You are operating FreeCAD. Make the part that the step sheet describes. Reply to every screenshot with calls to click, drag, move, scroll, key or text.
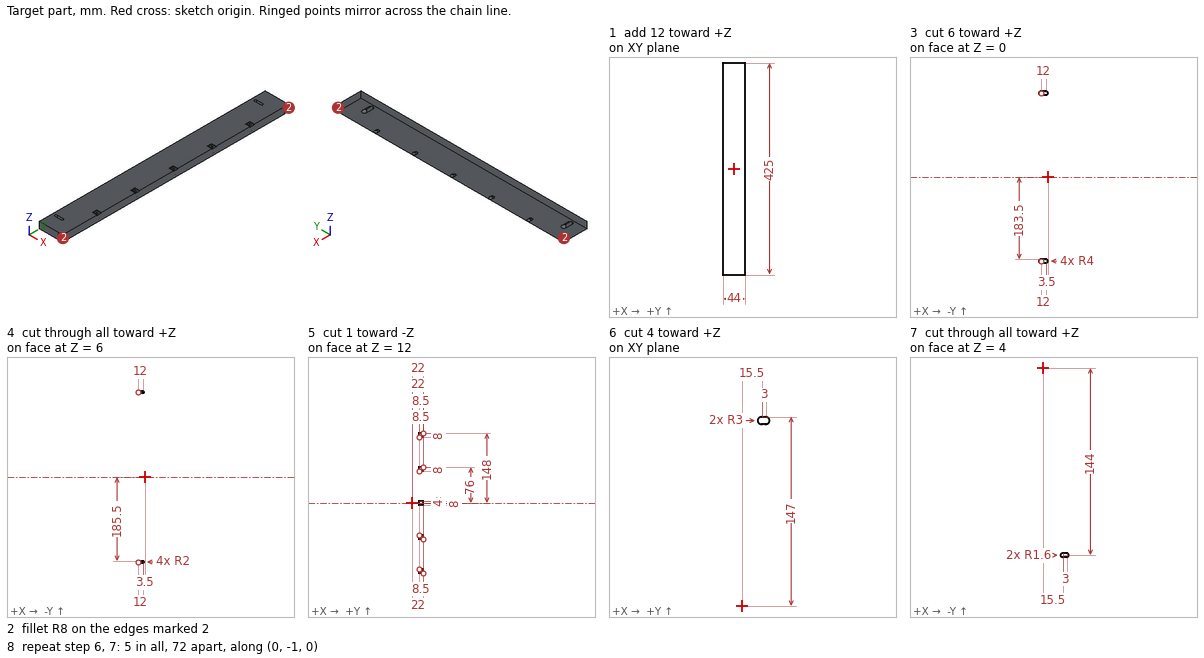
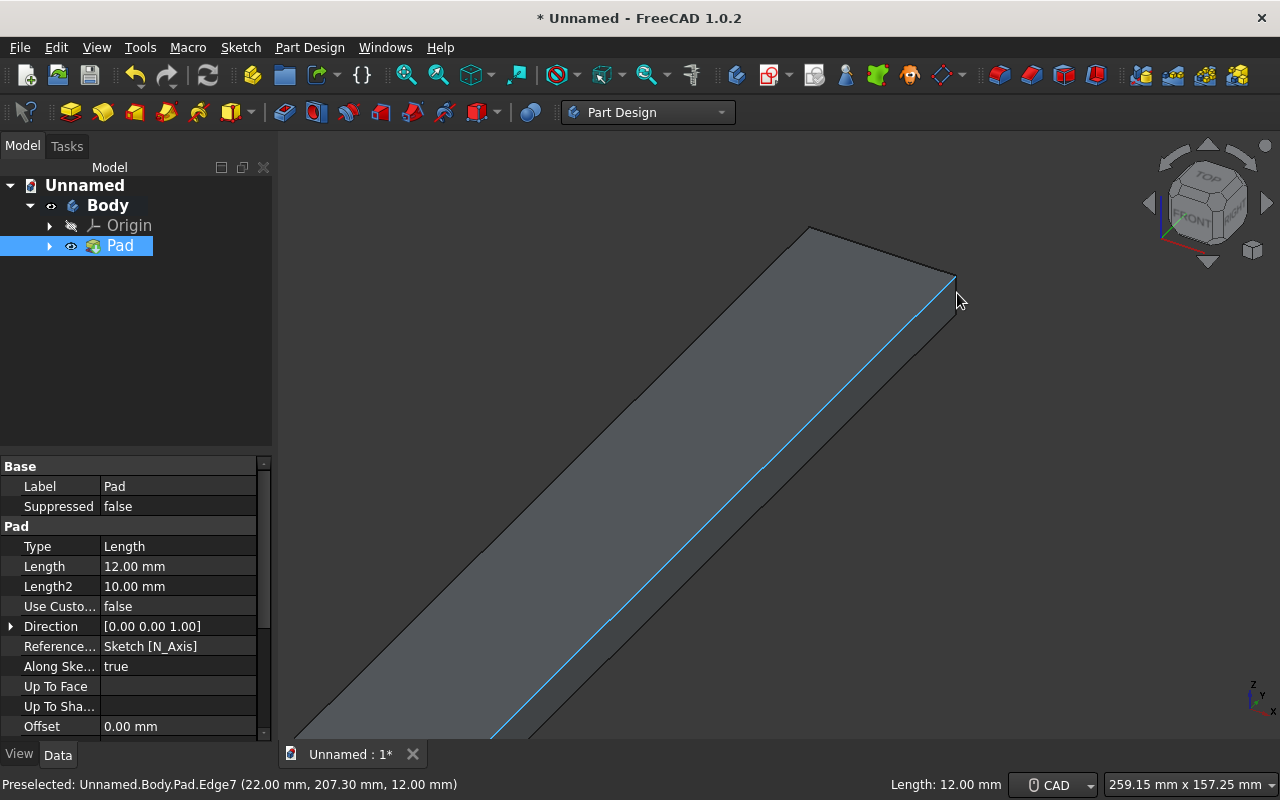
click(408, 76)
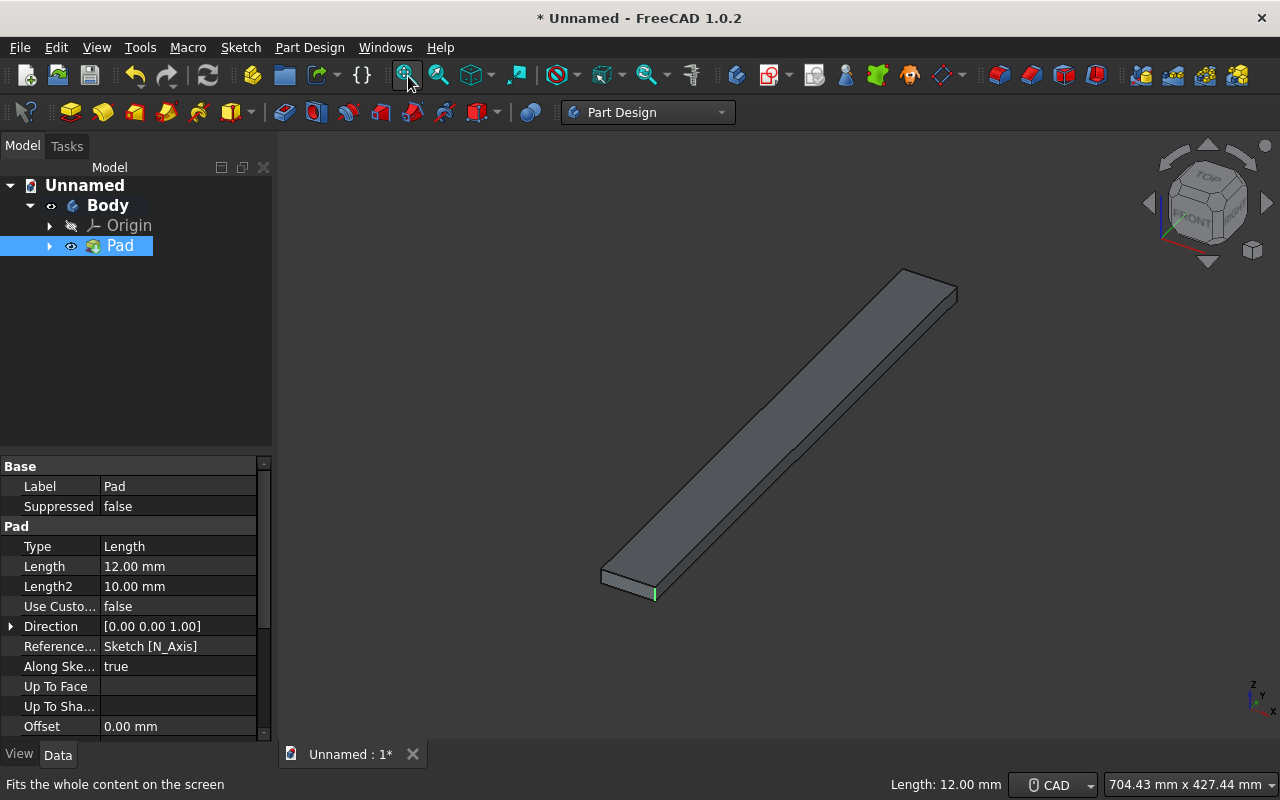
key(0)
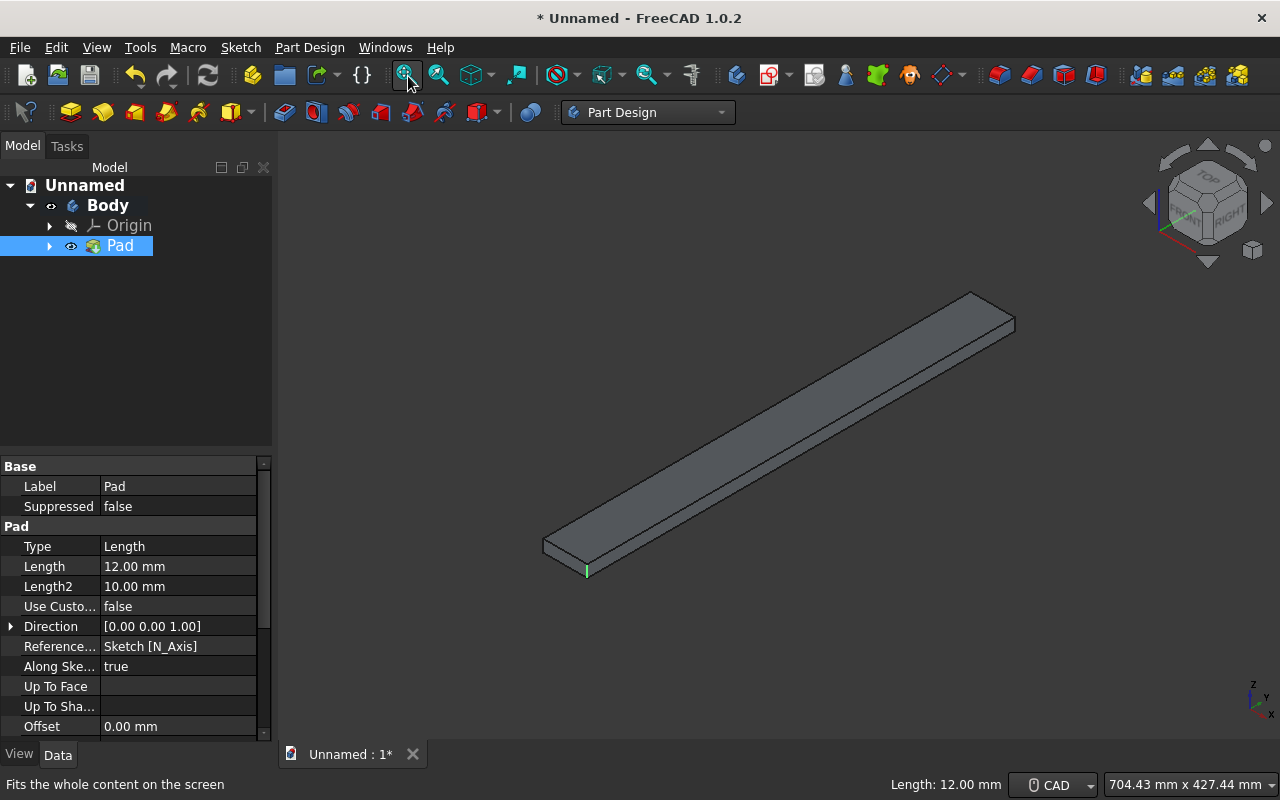
scroll(1015, 323, up, 5)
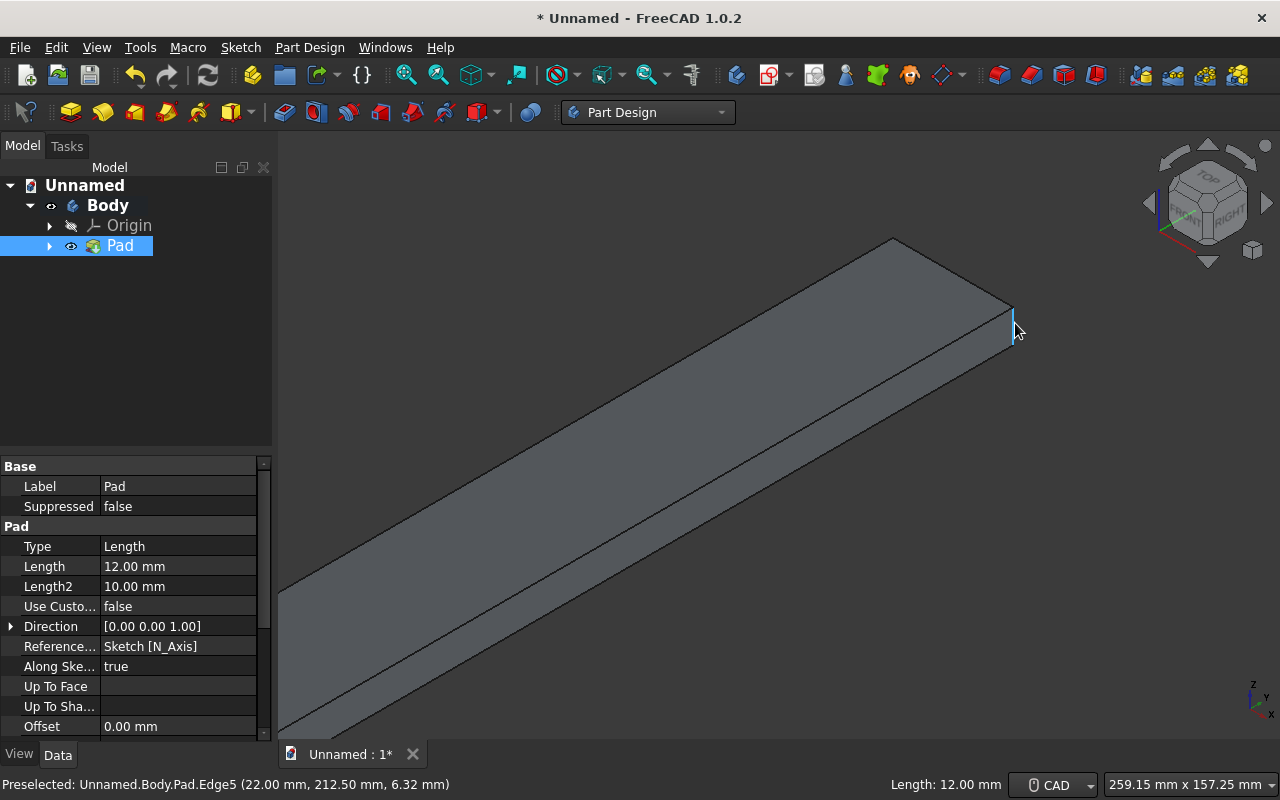
key(v)
key(f)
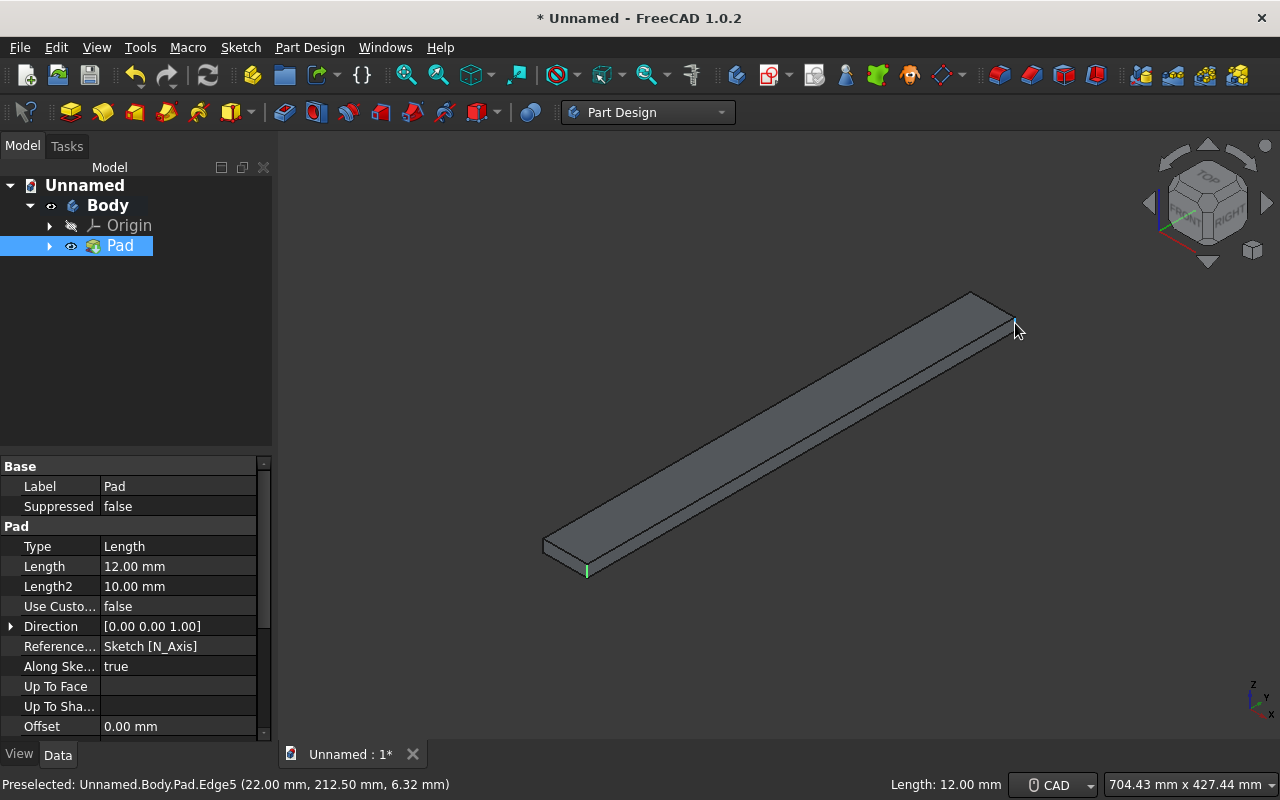
key(2)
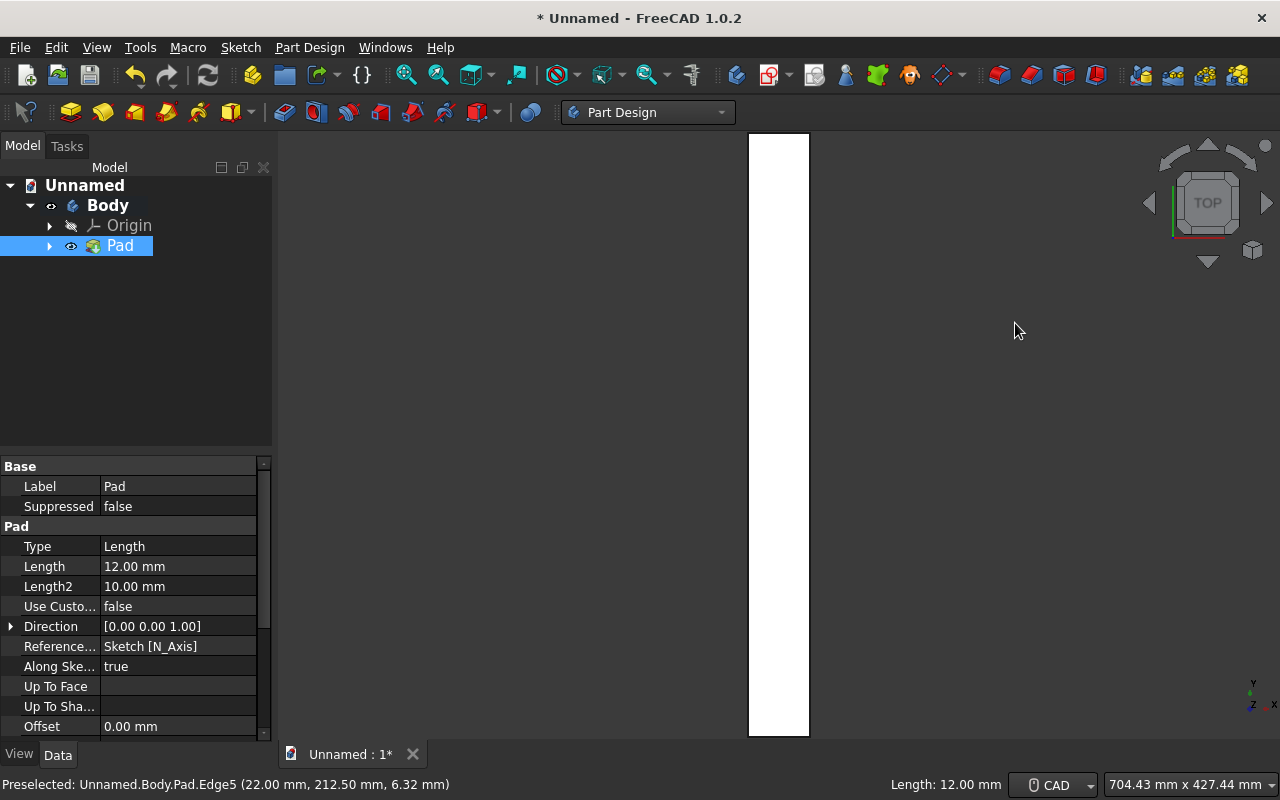
key(1)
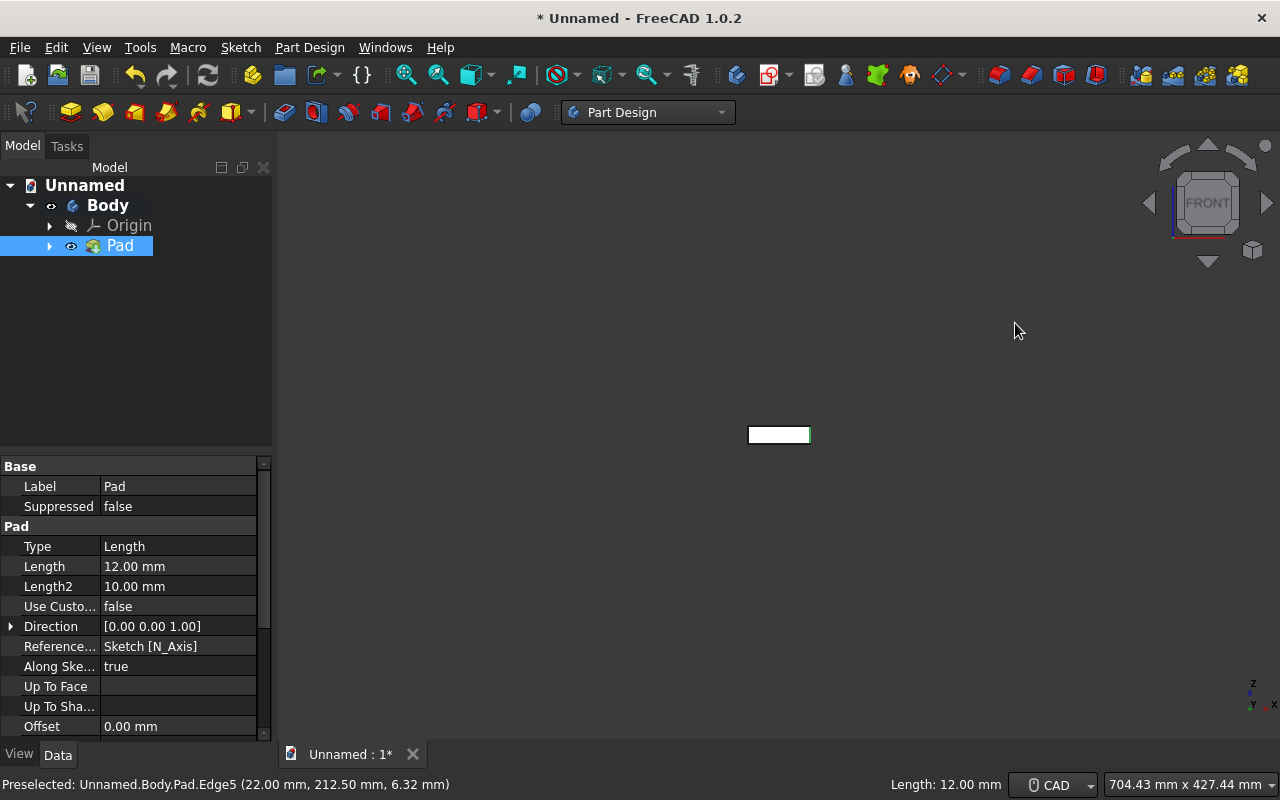
click(408, 76)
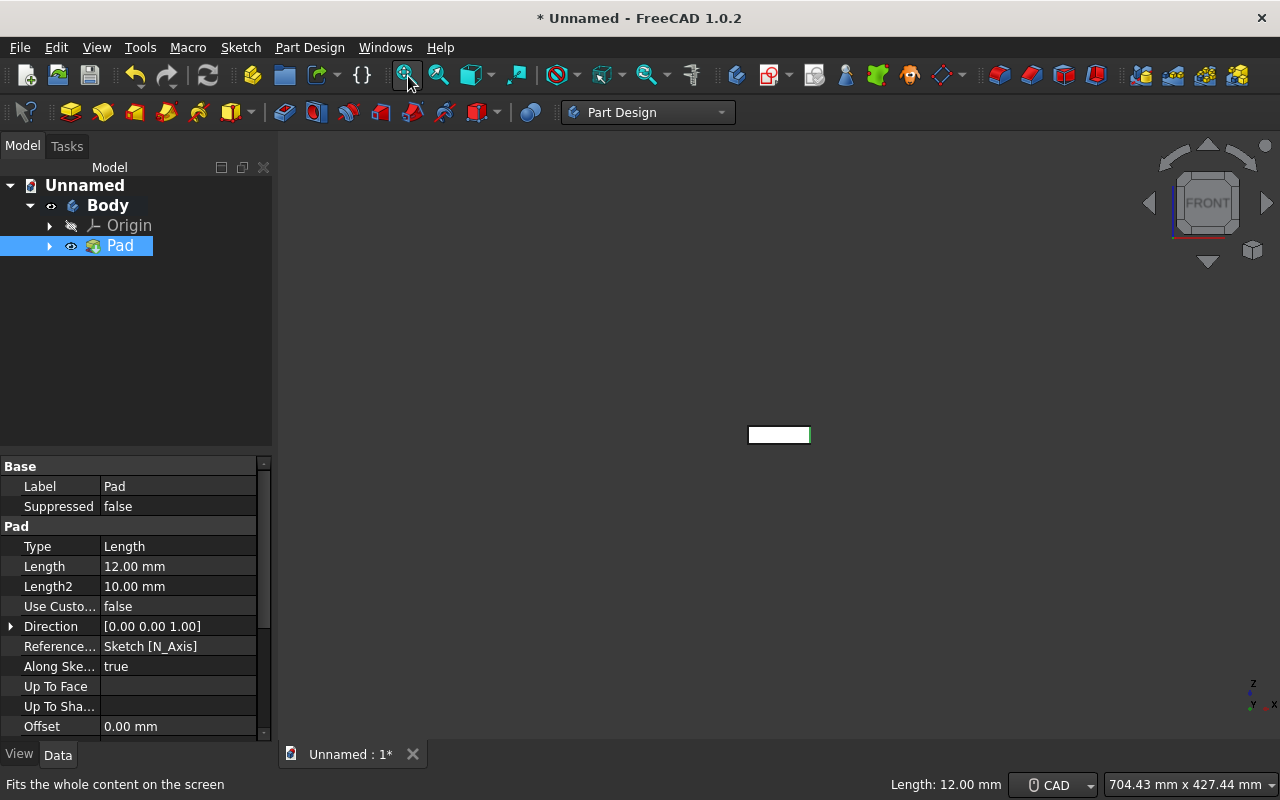
scroll(810, 434, up, 5)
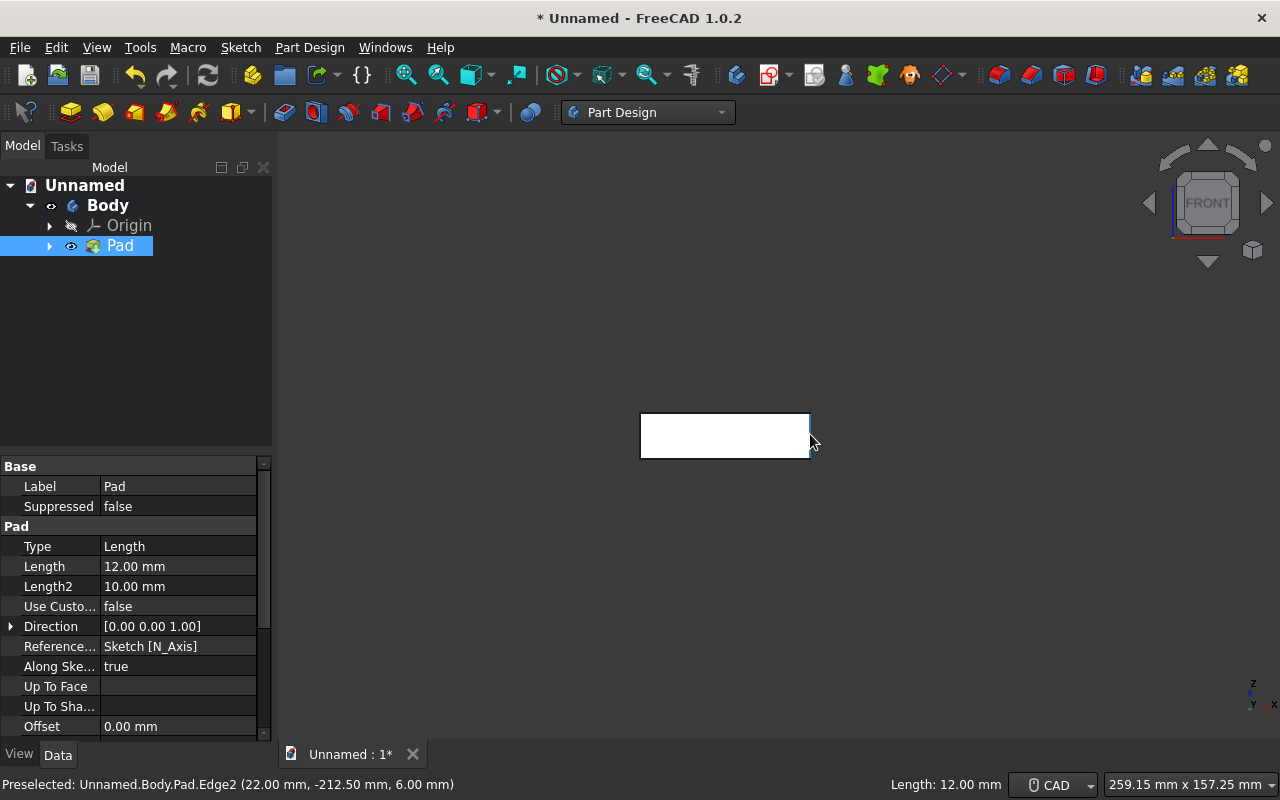
key(v)
key(f)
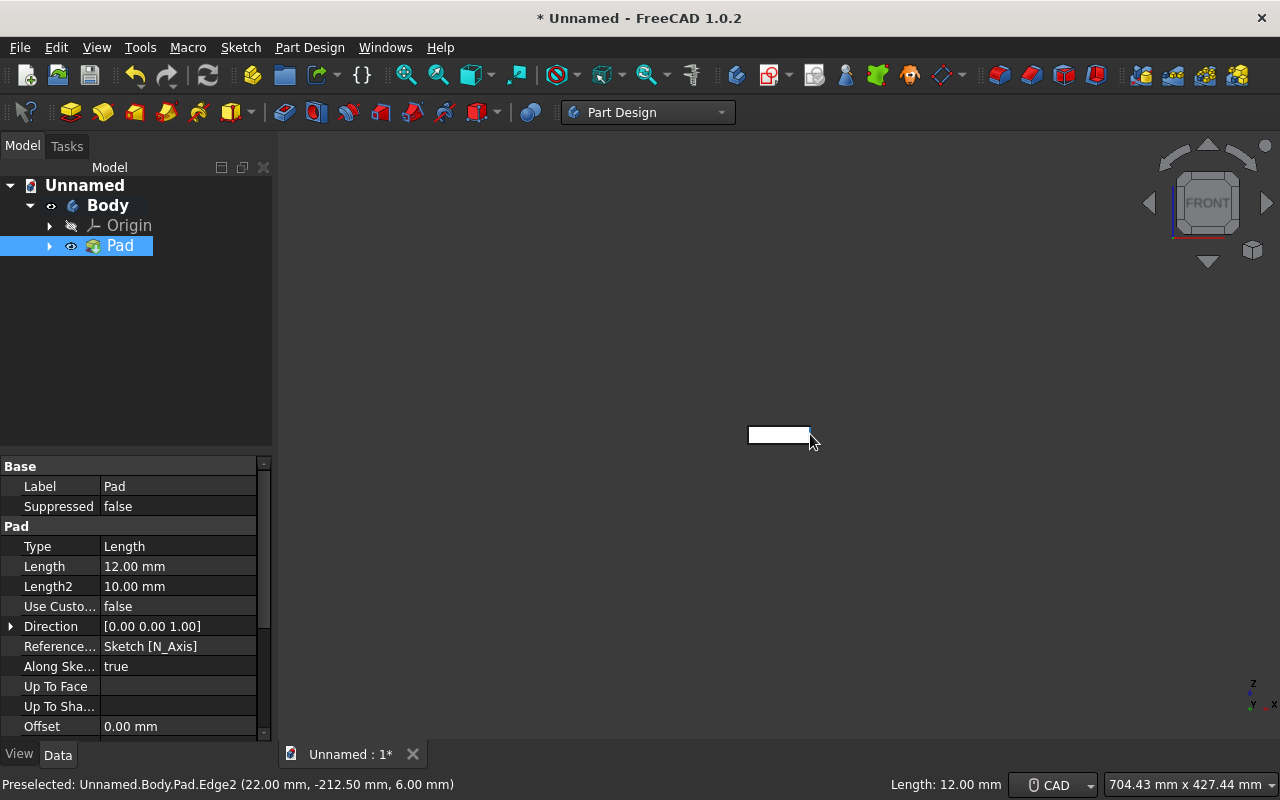
key(3)